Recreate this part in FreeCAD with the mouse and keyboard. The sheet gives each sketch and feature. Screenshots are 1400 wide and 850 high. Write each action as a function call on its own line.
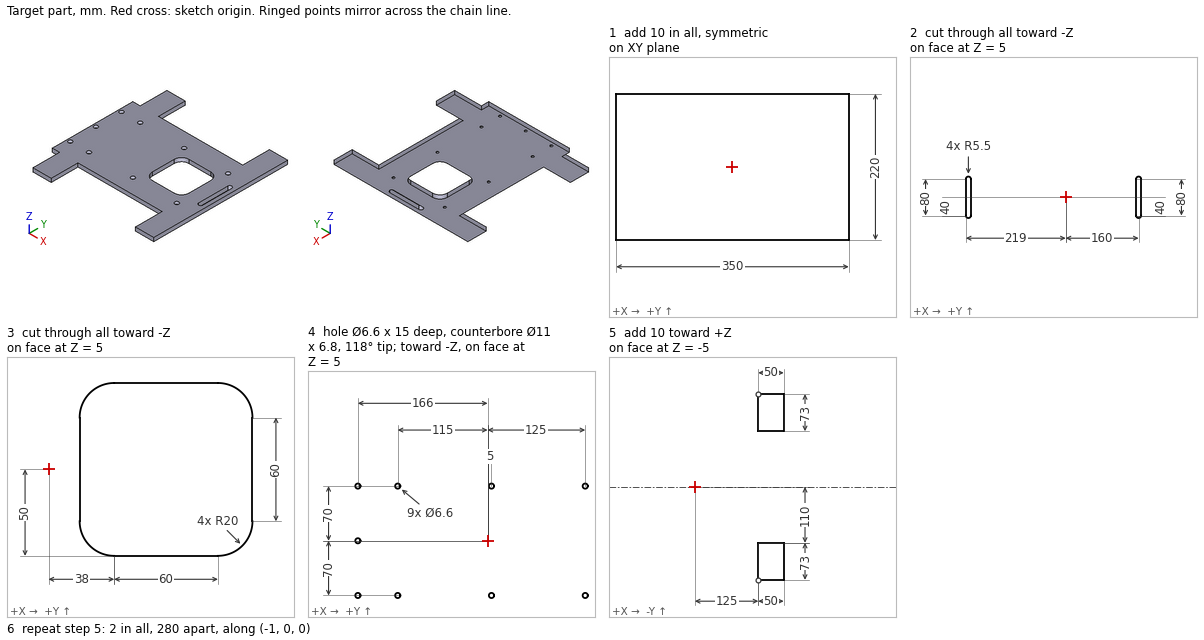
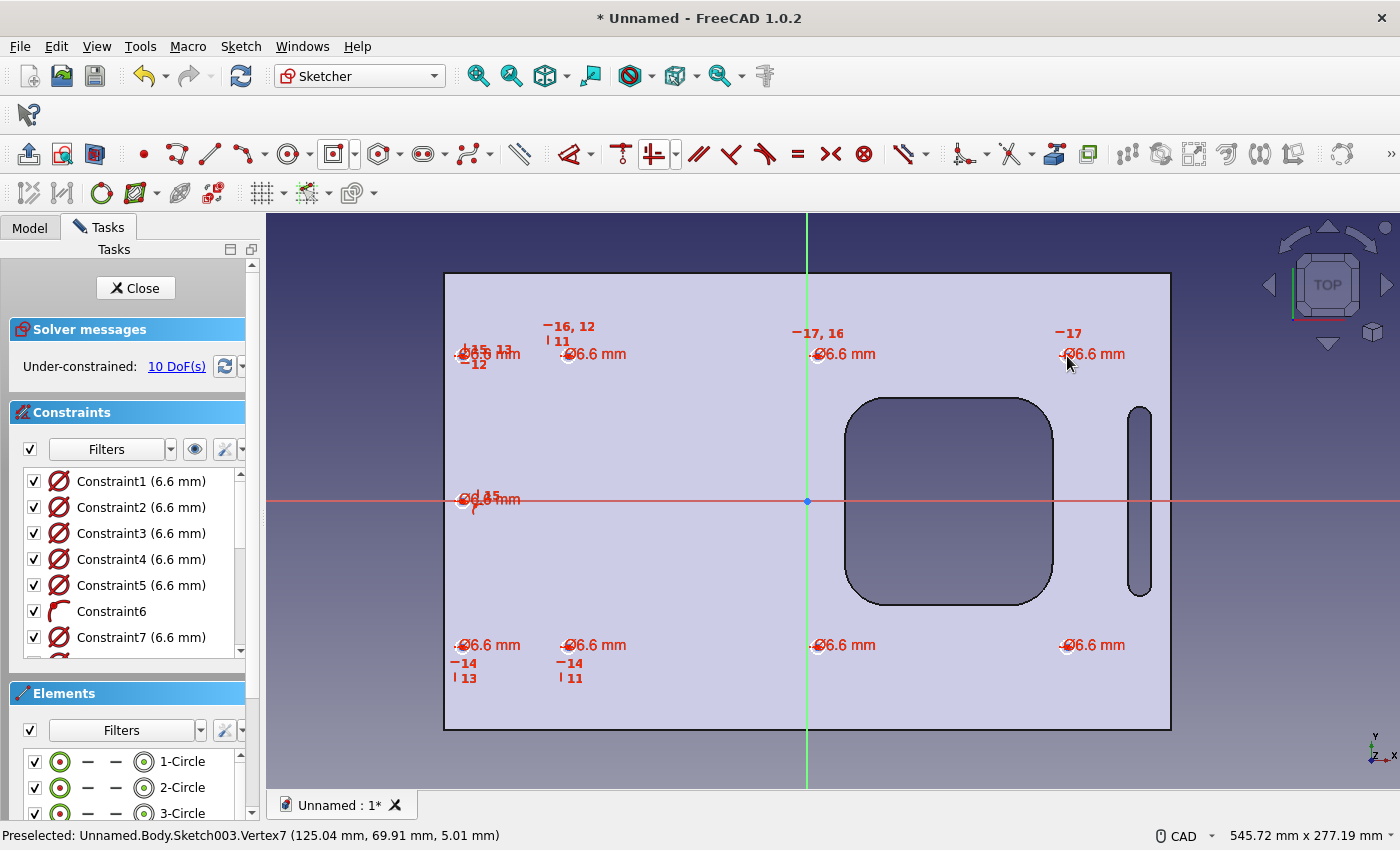
click(1067, 356)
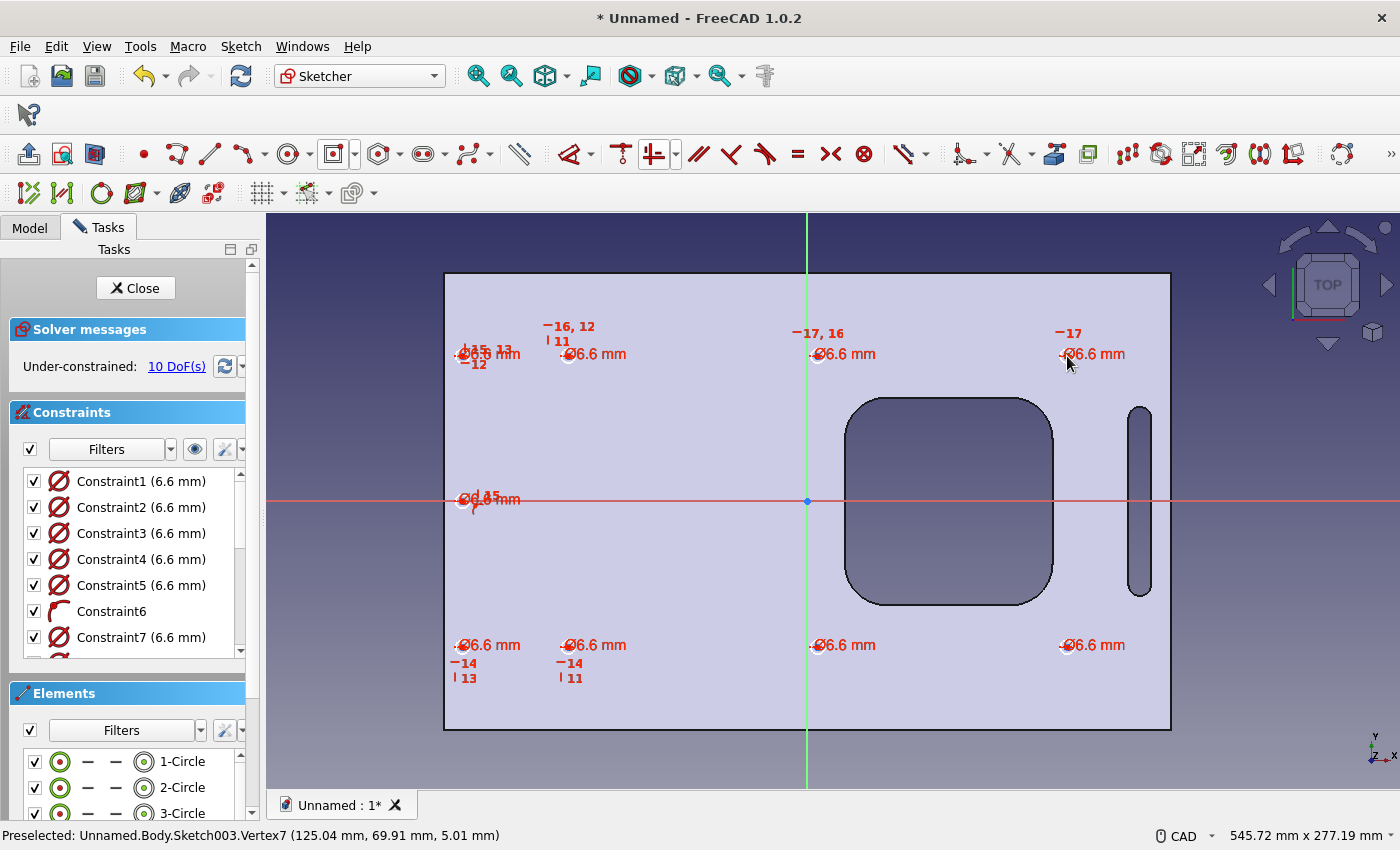
click(1067, 647)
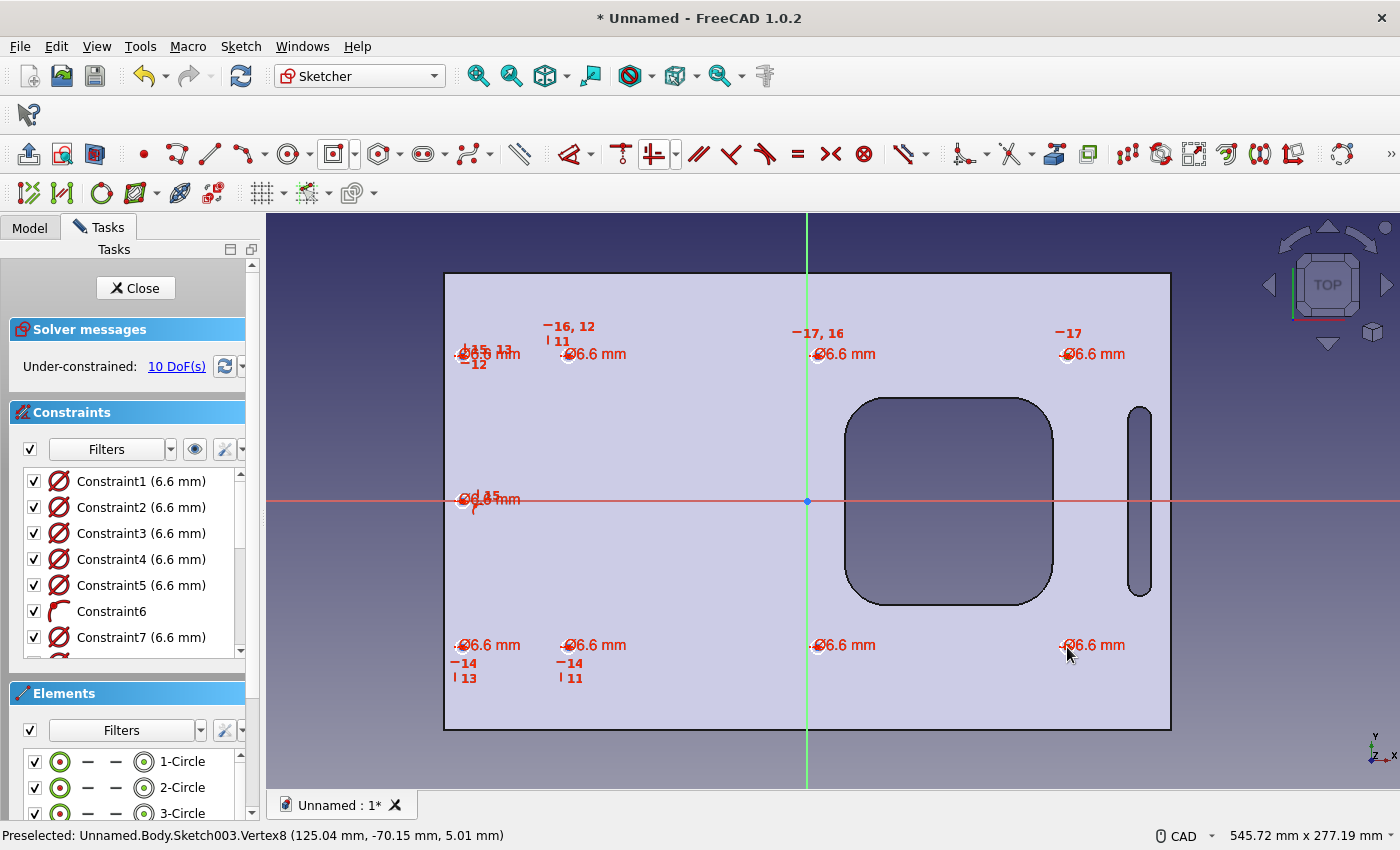
click(676, 154)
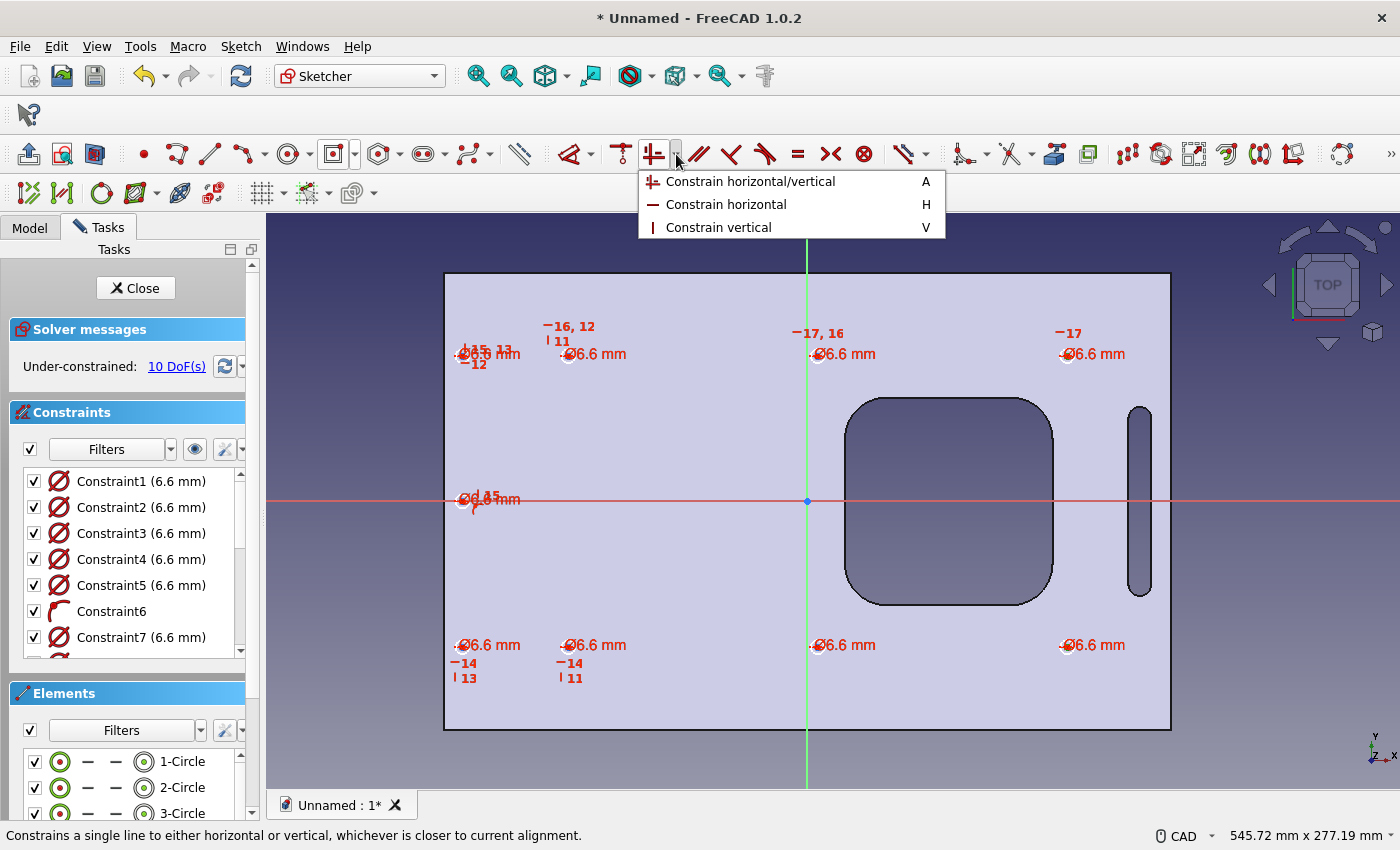
click(792, 228)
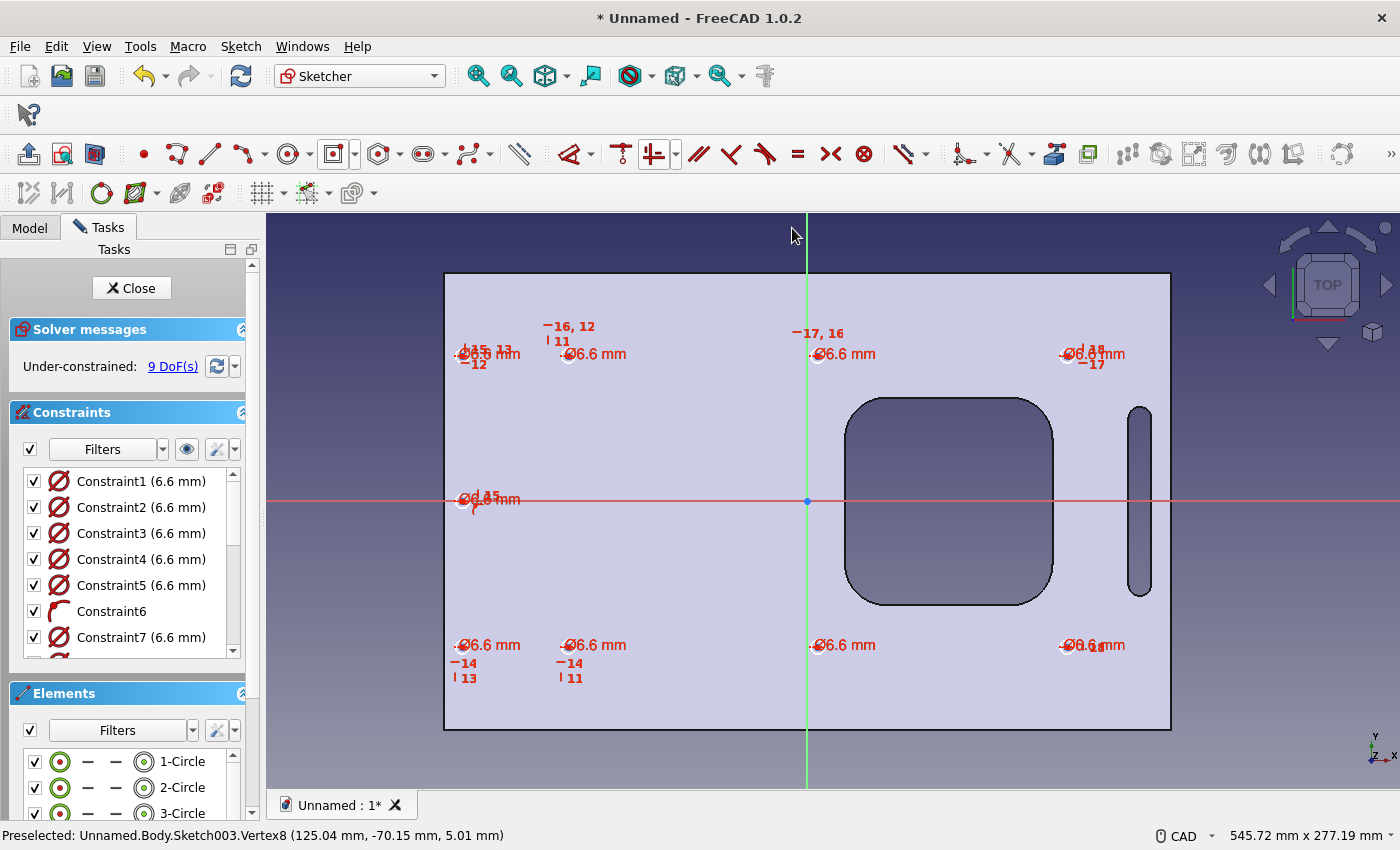
click(568, 647)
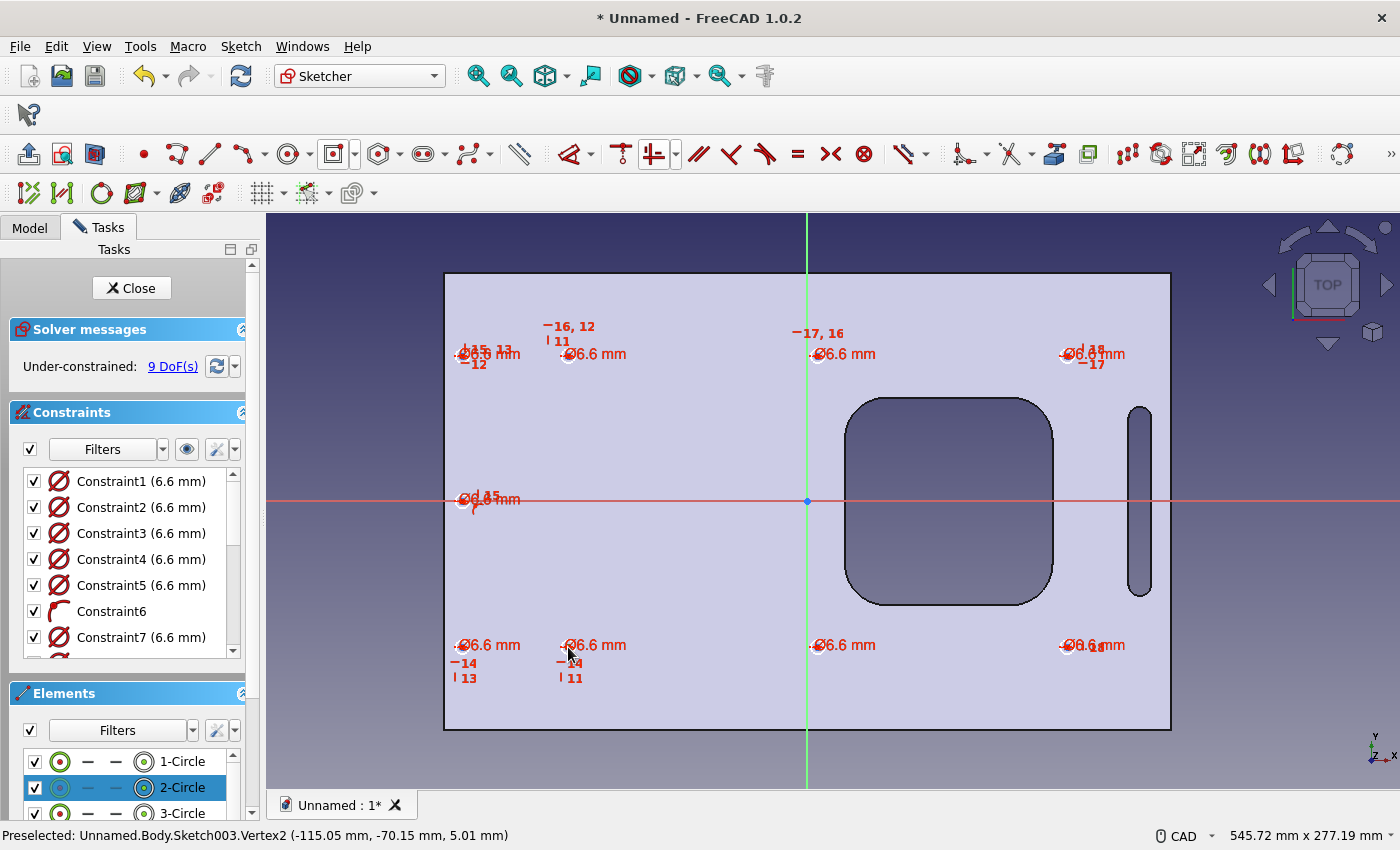
click(1067, 647)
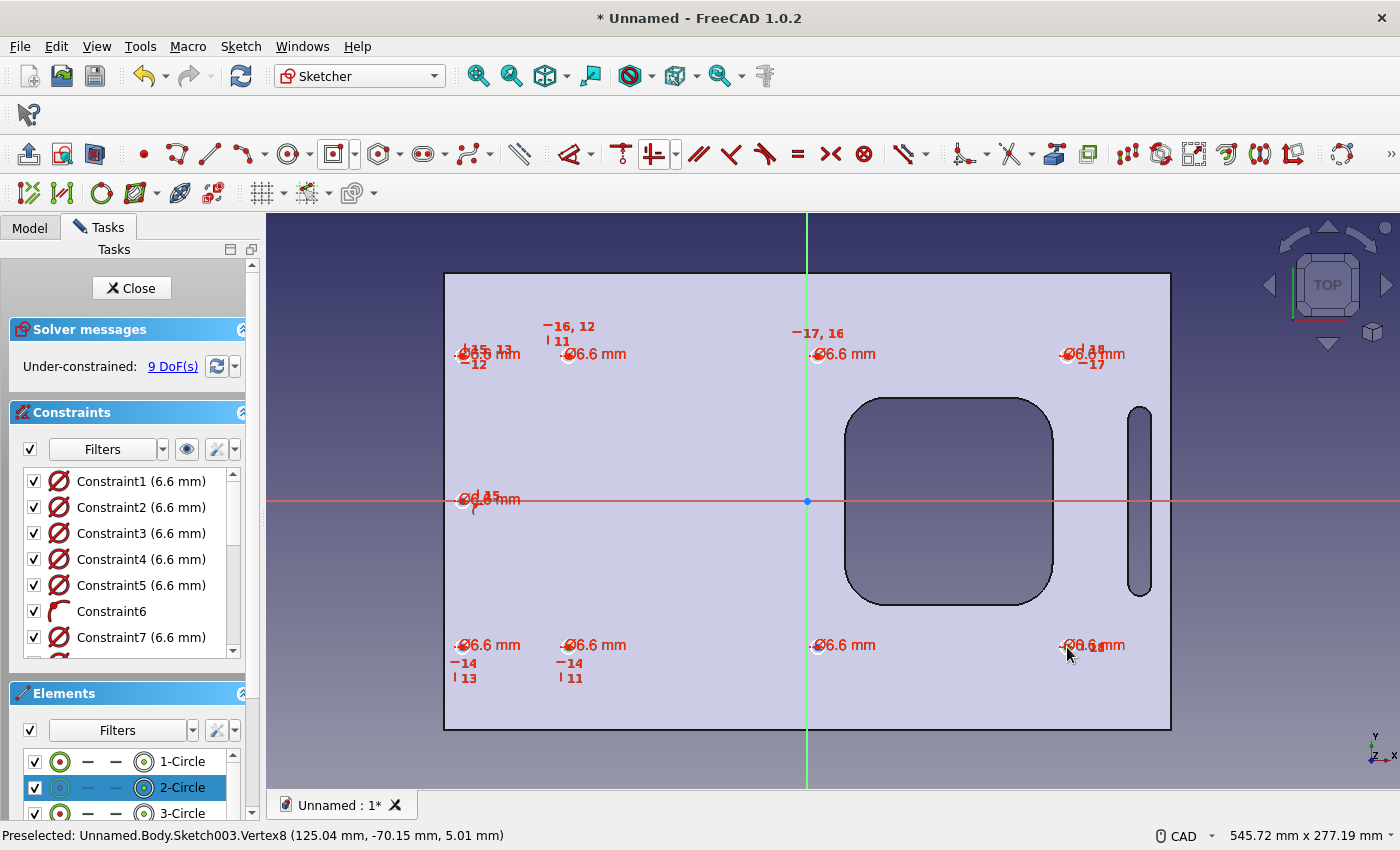
key(h)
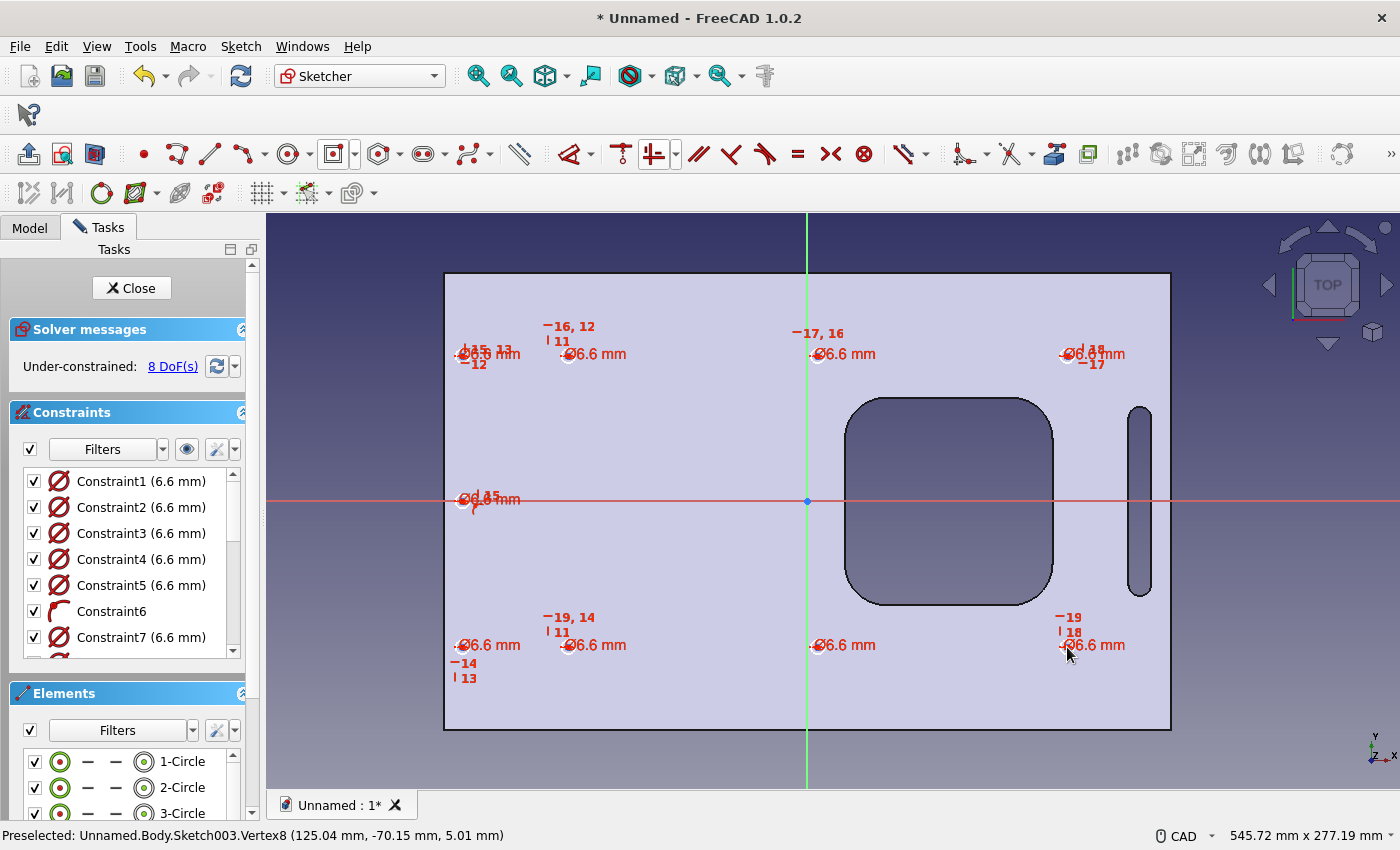
click(818, 356)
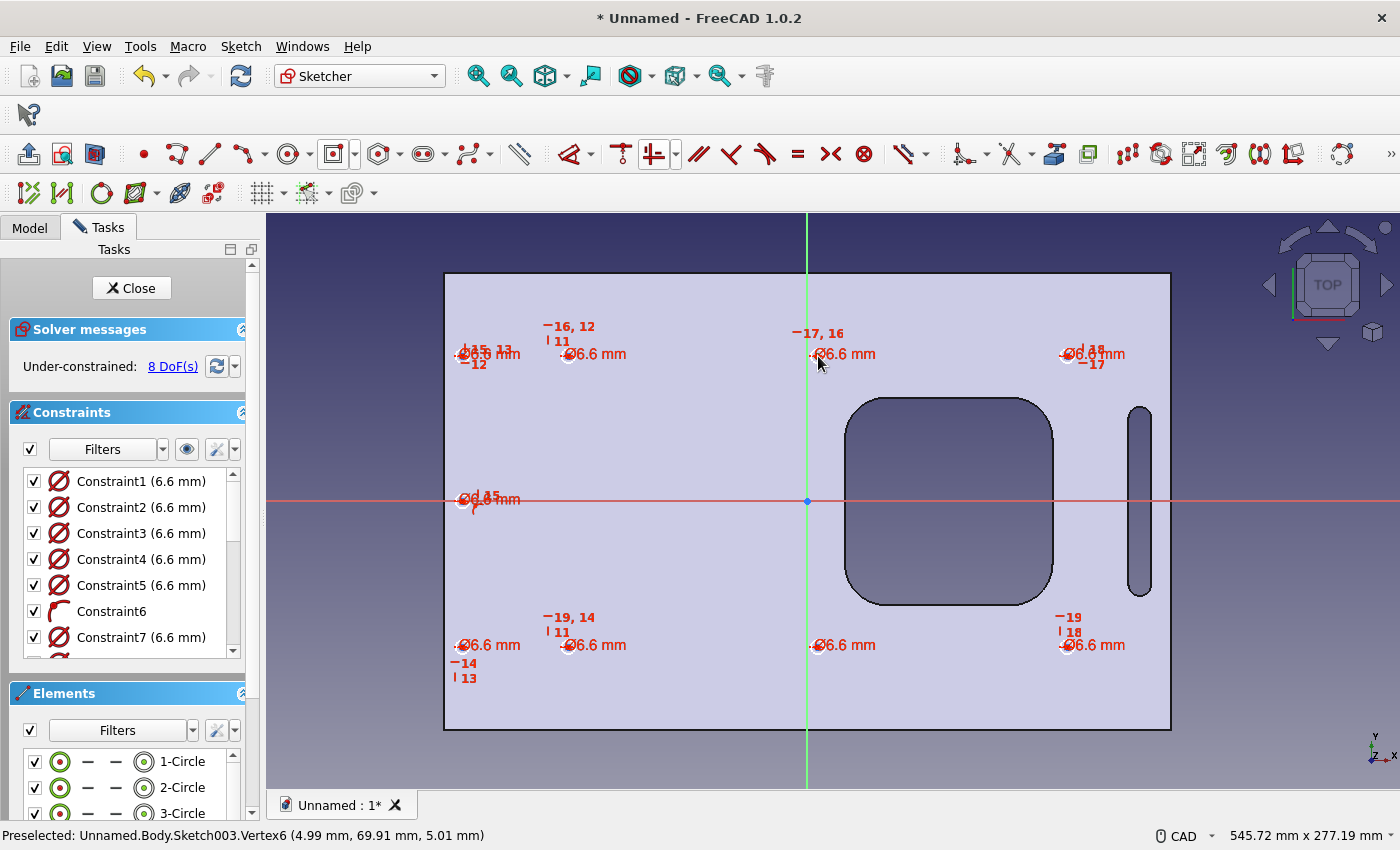
click(818, 647)